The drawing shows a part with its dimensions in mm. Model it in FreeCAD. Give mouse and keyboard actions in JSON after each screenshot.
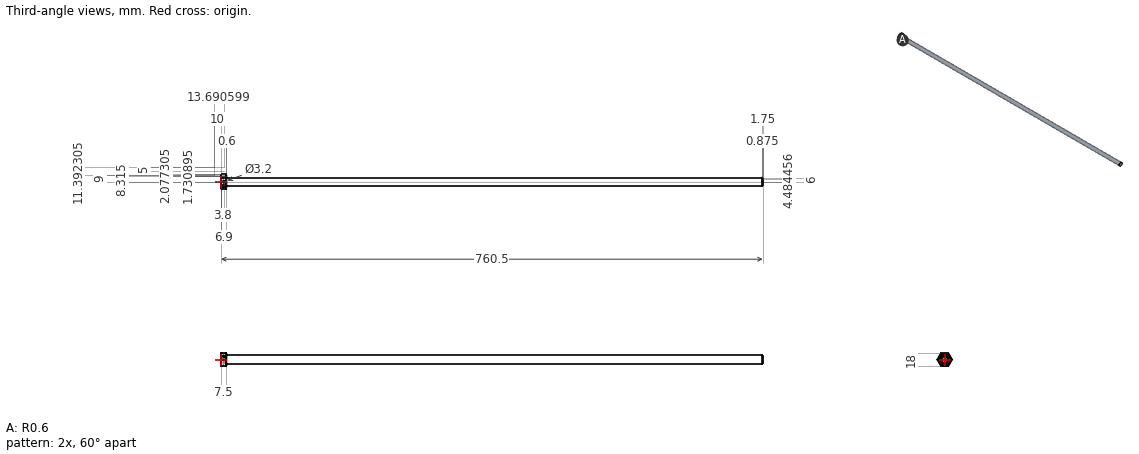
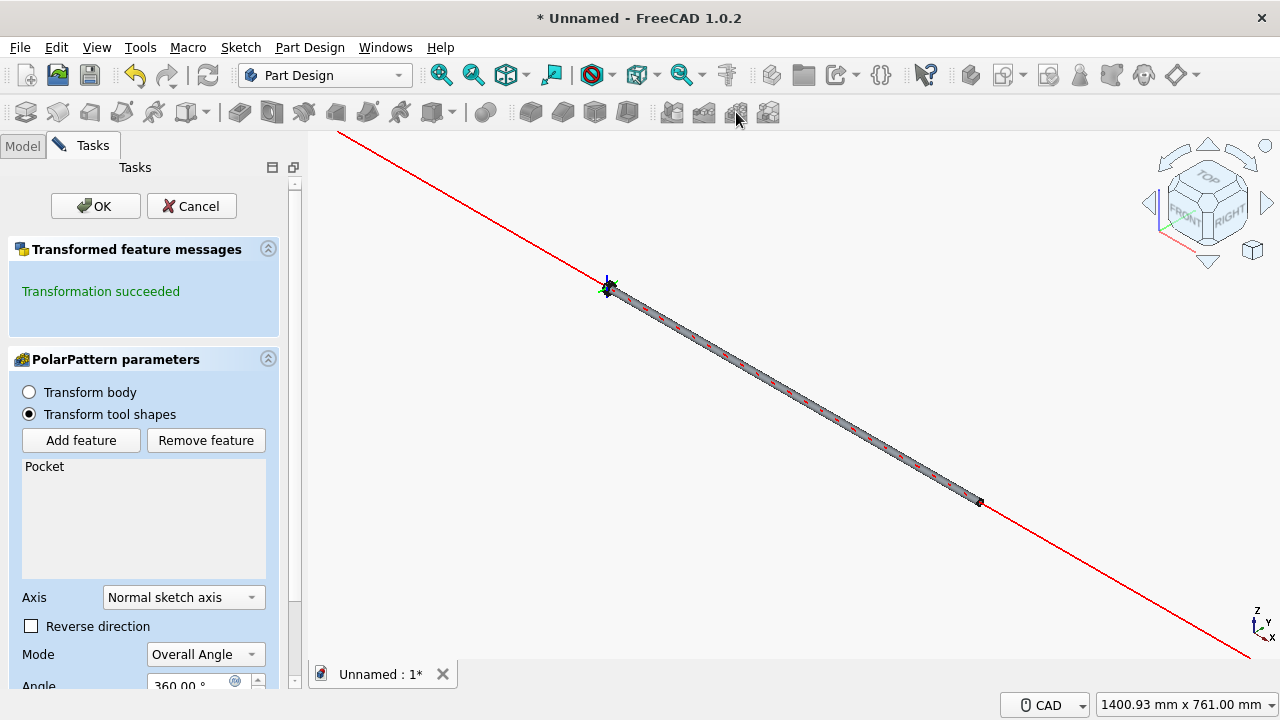
{"action": "left_click", "coordinate": [184, 598]}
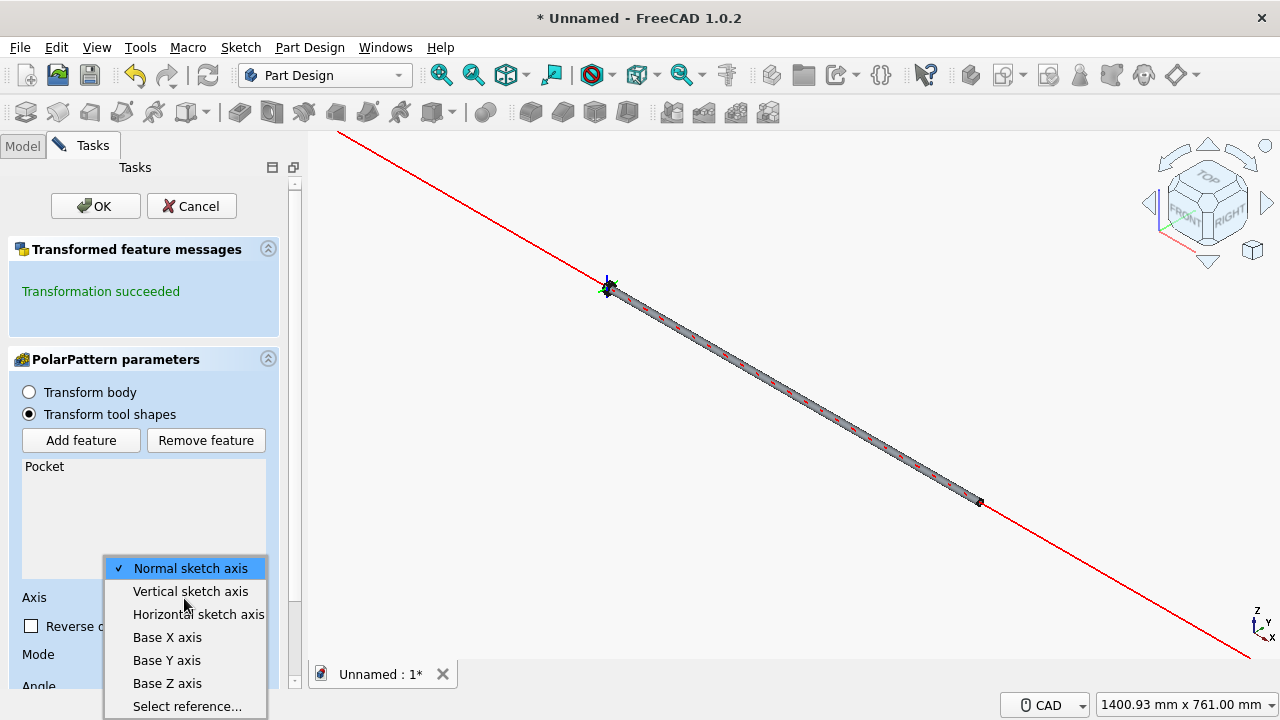
{"action": "left_click", "coordinate": [184, 638]}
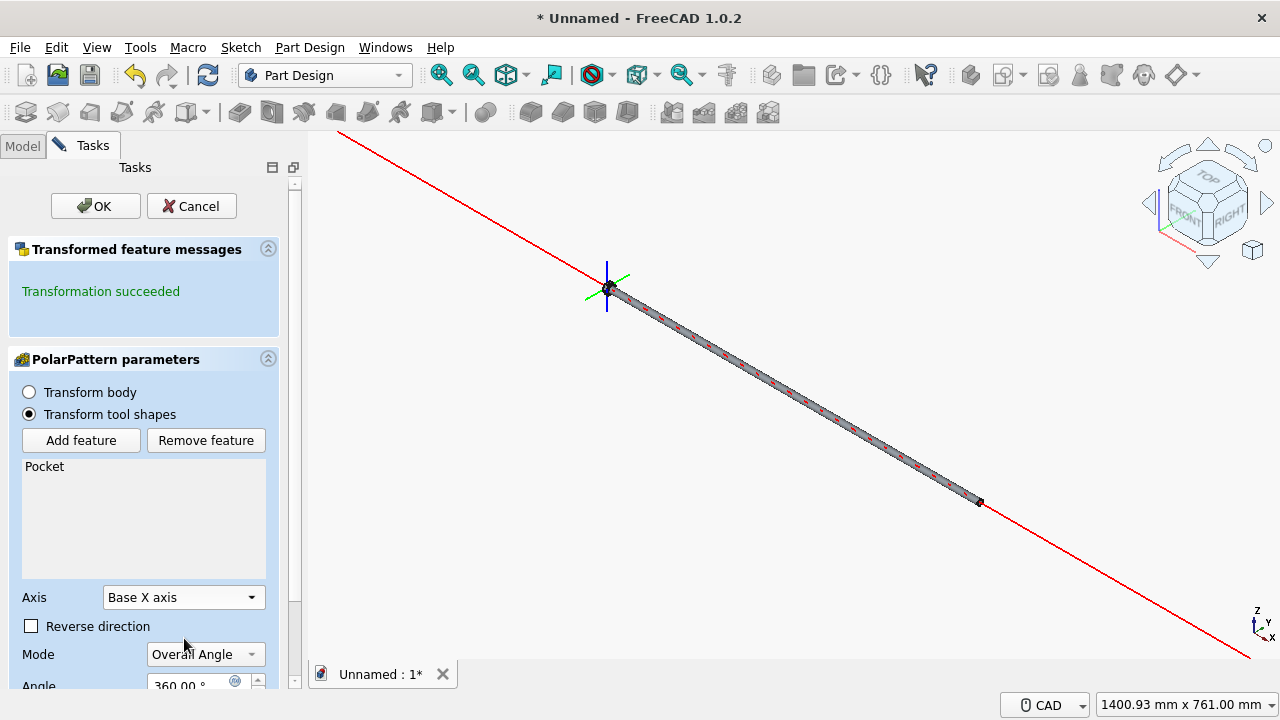
{"action": "left_click", "coordinate": [206, 654]}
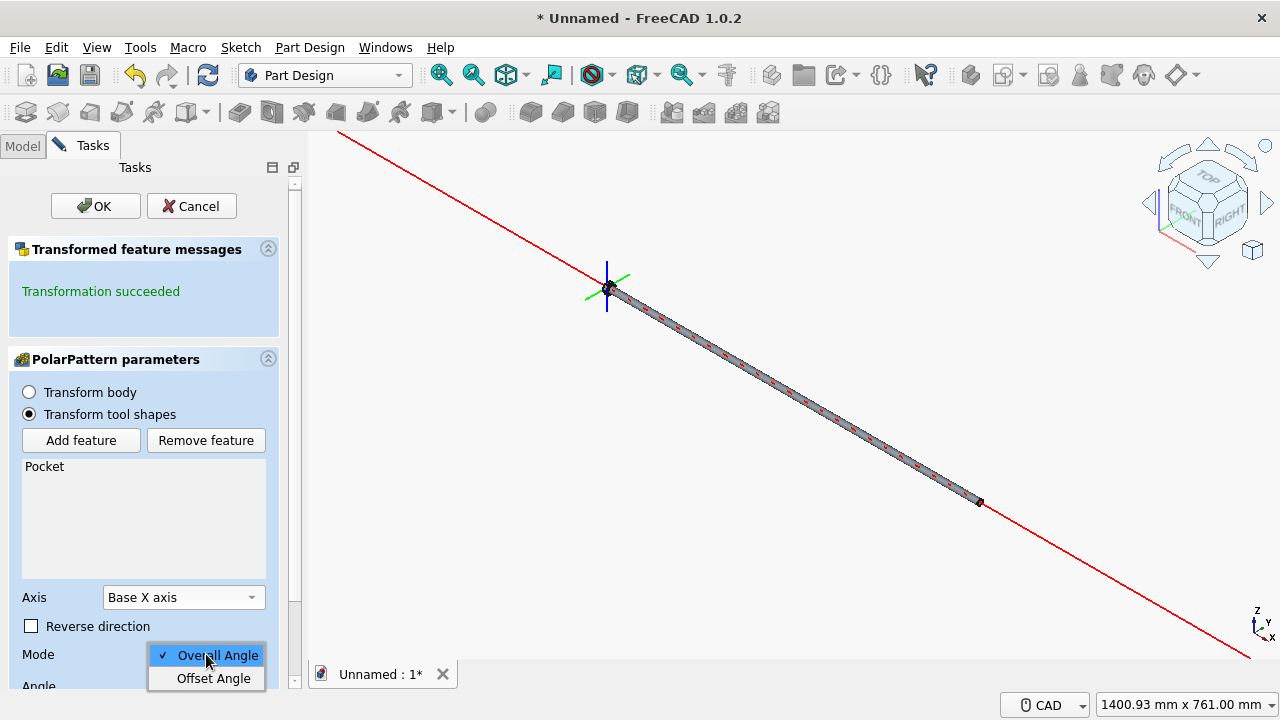
{"action": "left_click", "coordinate": [206, 678]}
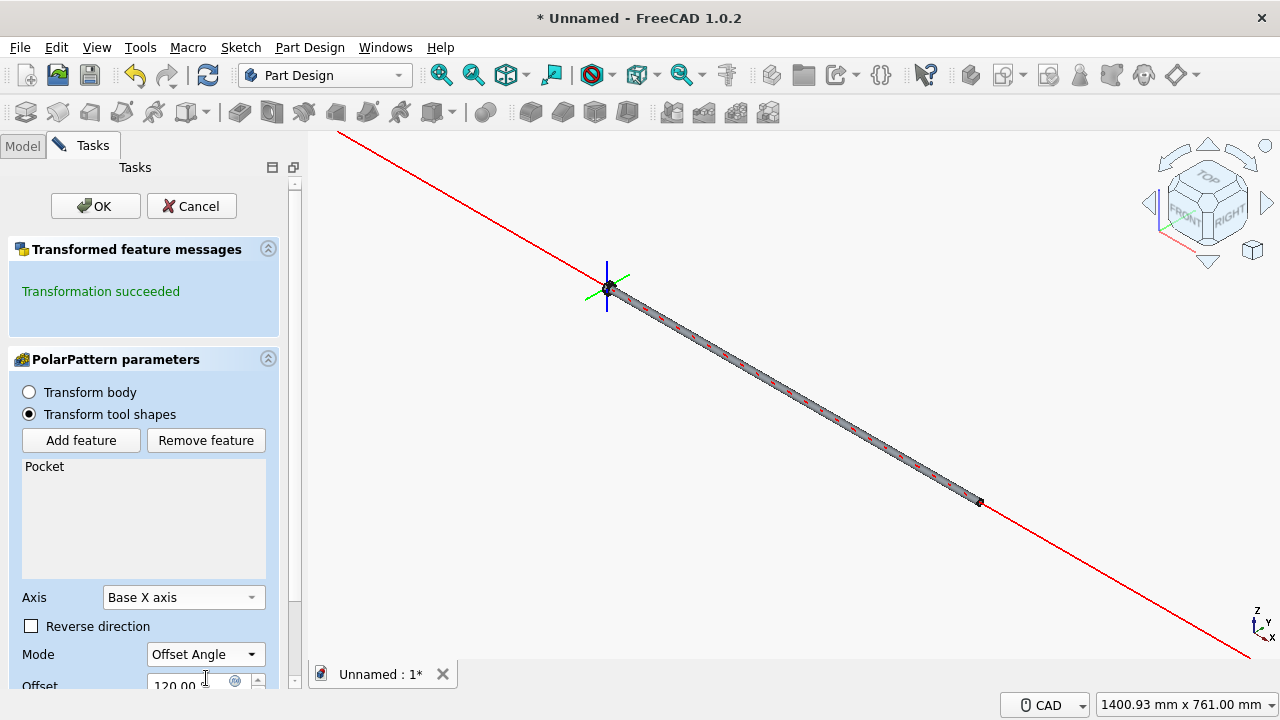
{"action": "scroll", "coordinate": [295, 432], "scroll_direction": "down", "scroll_amount": 2}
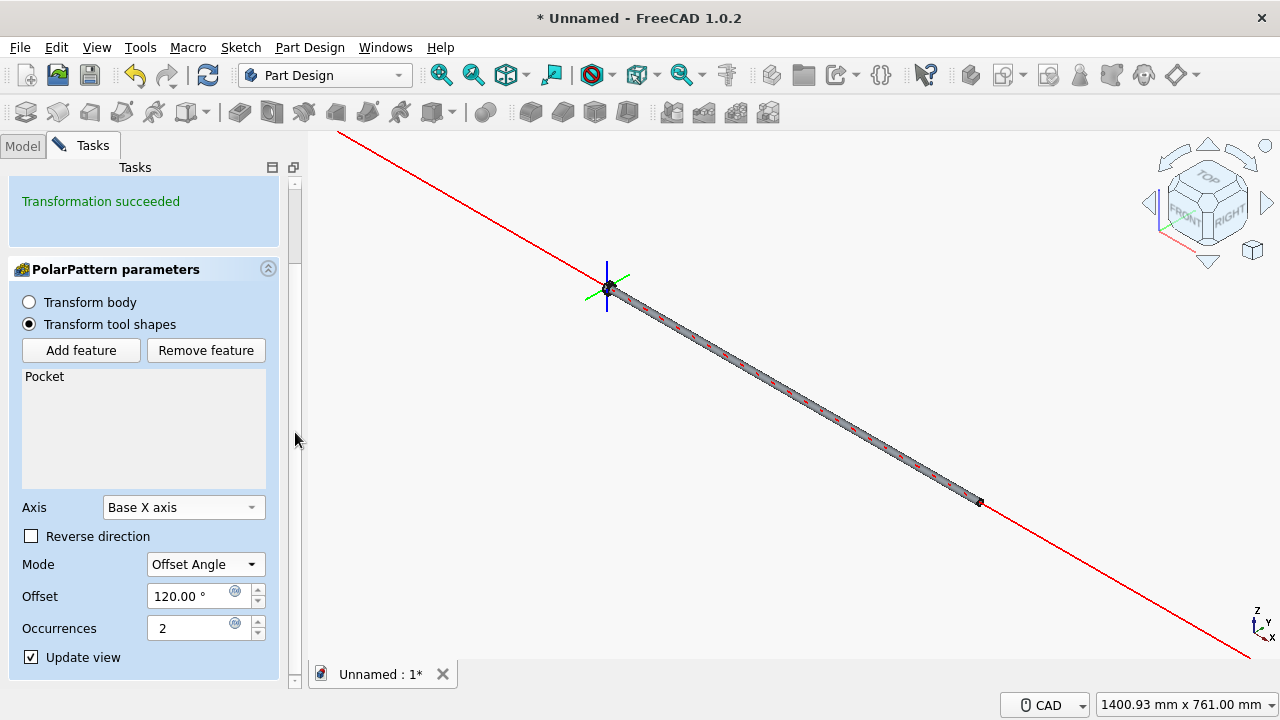
{"action": "triple_click", "coordinate": [198, 596]}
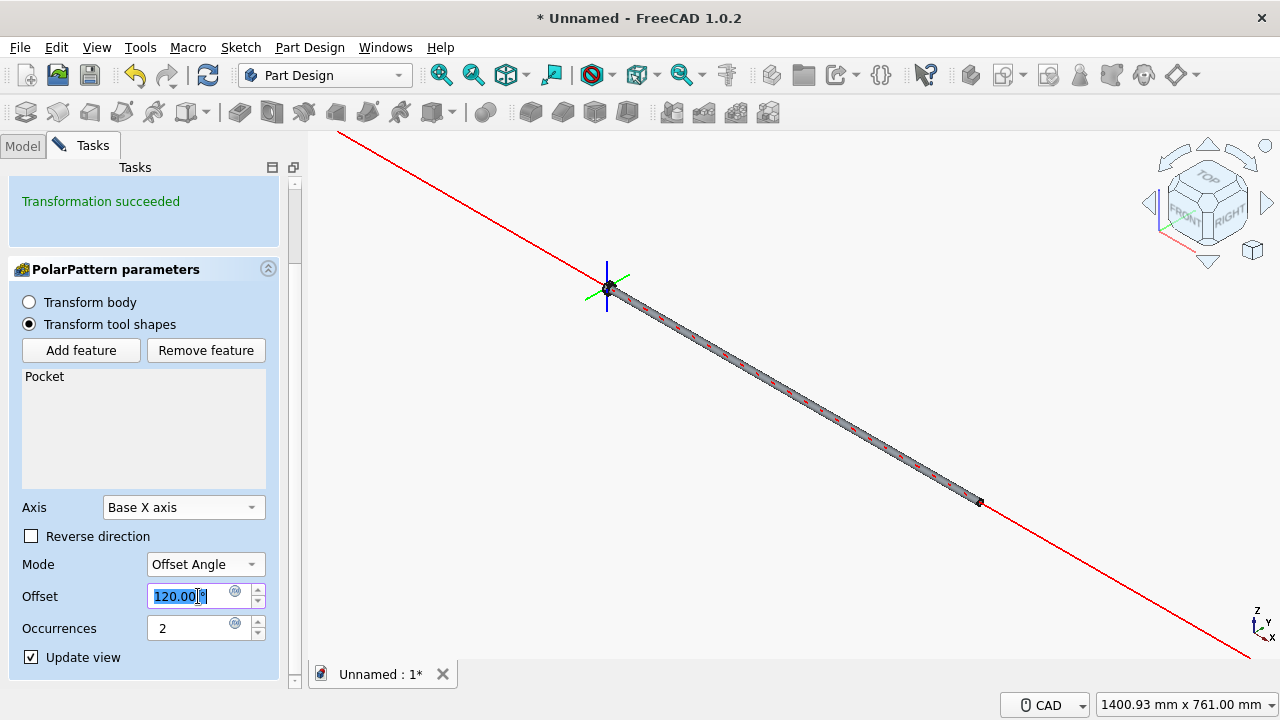
{"action": "type", "text": "60"}
{"action": "key", "text": "Tab"}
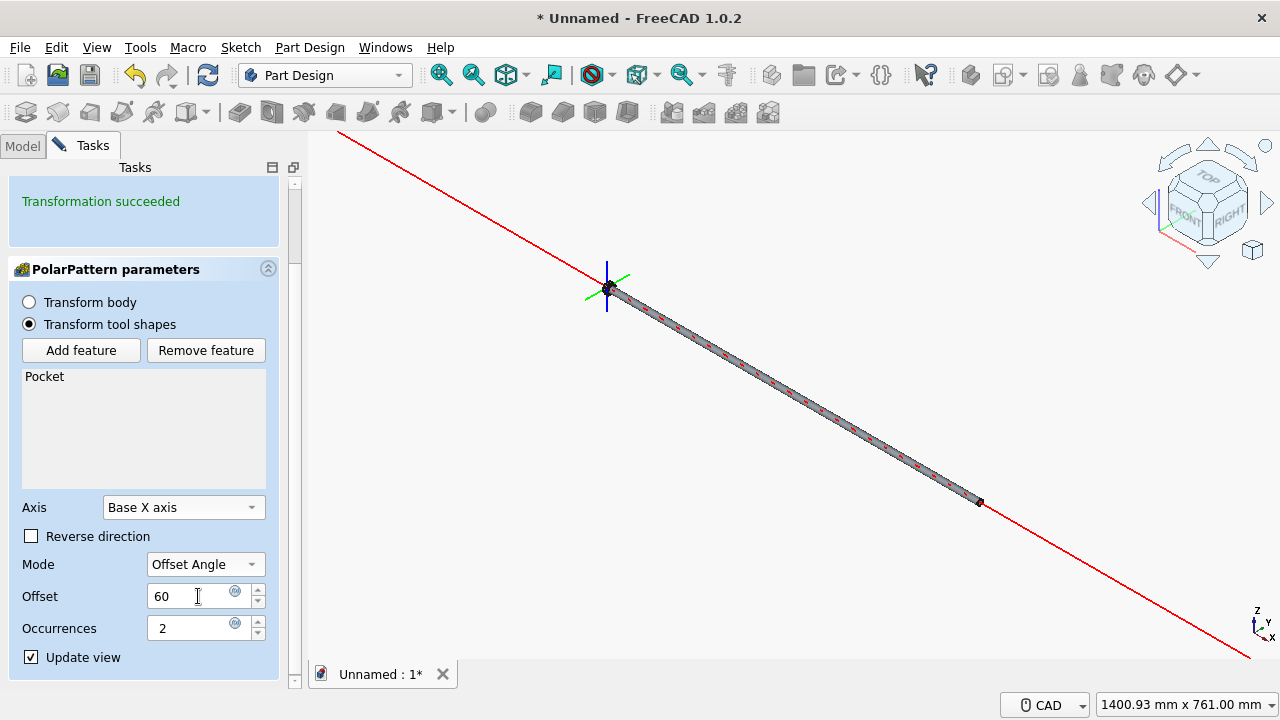
{"action": "triple_click", "coordinate": [198, 628]}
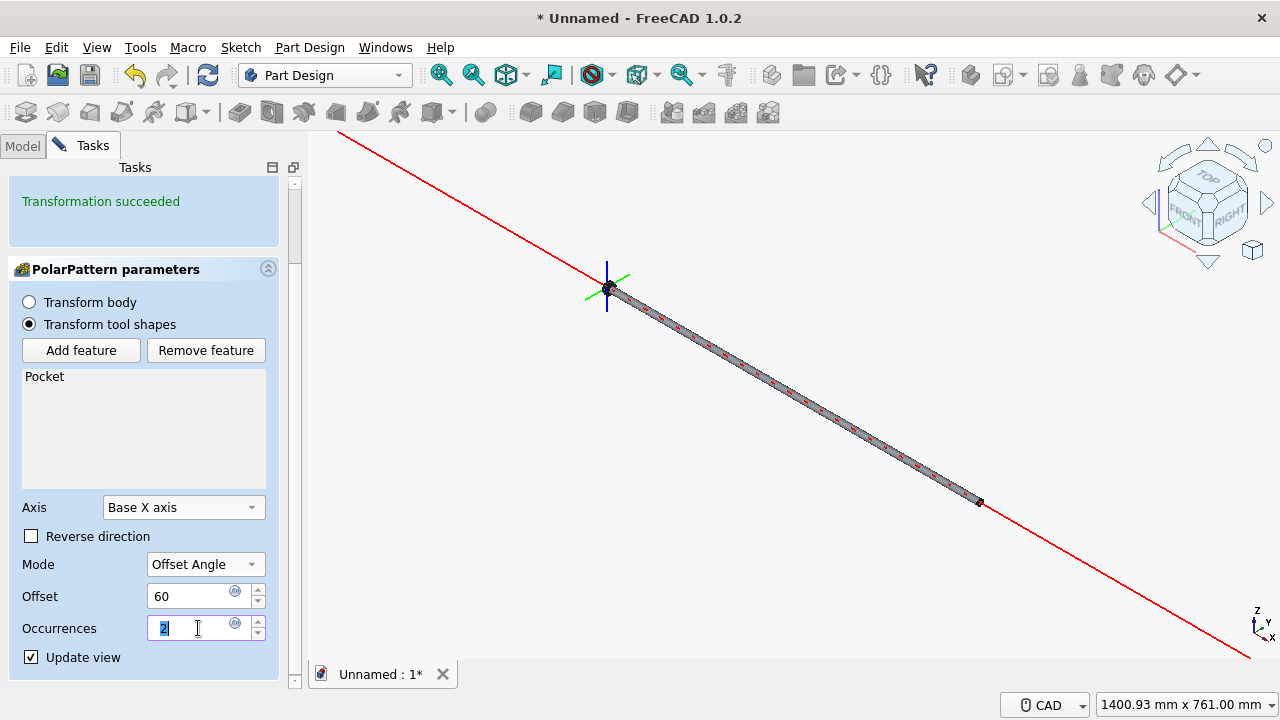
{"action": "type", "text": "2"}
{"action": "key", "text": "Tab"}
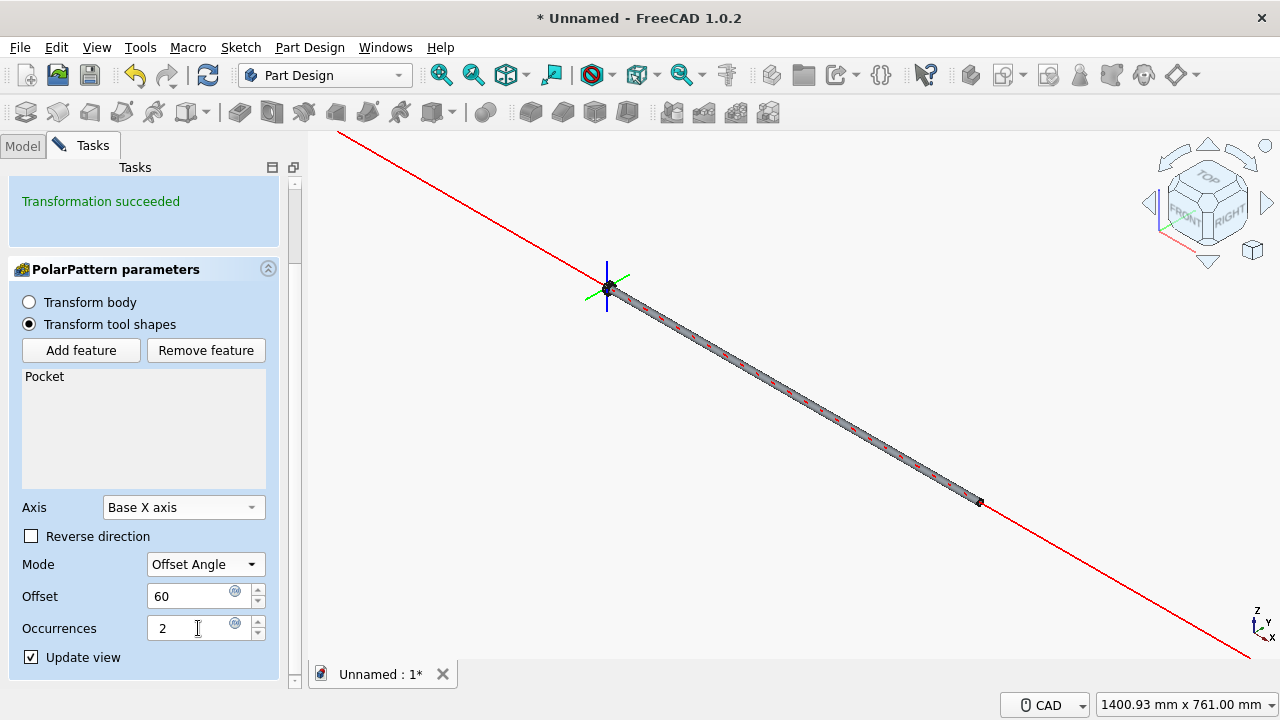
{"action": "scroll", "coordinate": [295, 432], "scroll_direction": "up", "scroll_amount": 3}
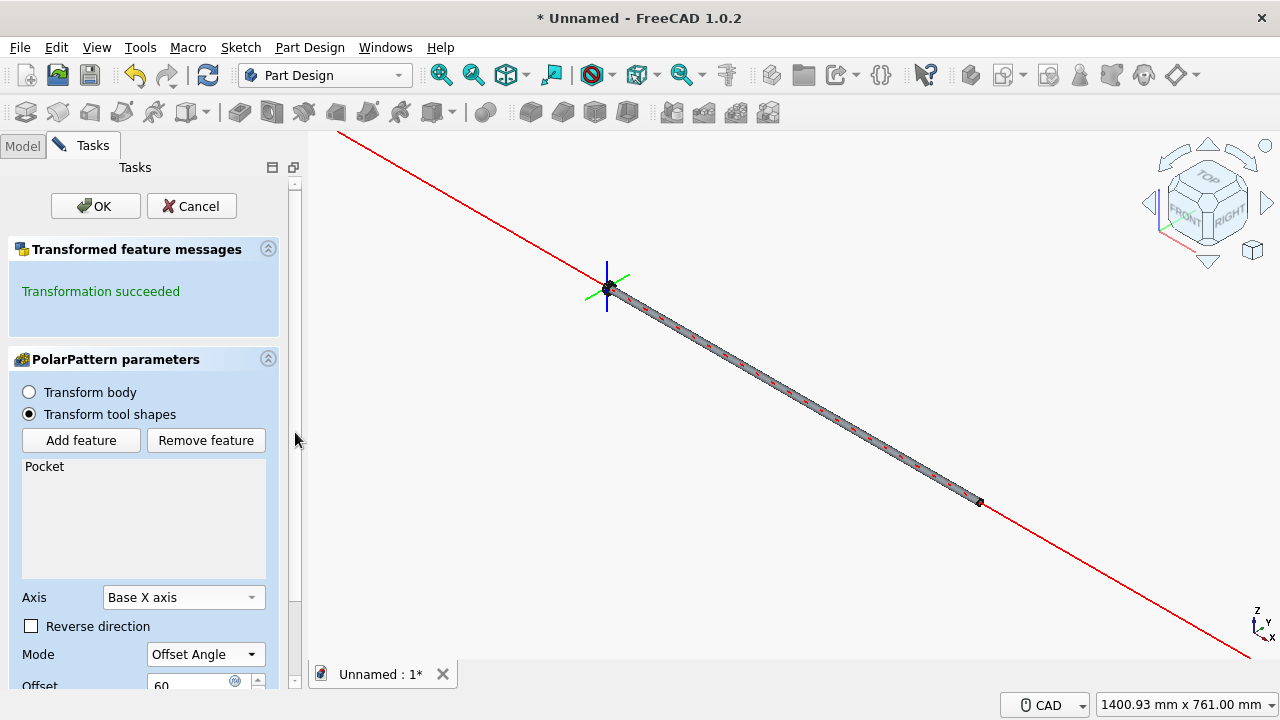
{"action": "left_click", "coordinate": [96, 206]}